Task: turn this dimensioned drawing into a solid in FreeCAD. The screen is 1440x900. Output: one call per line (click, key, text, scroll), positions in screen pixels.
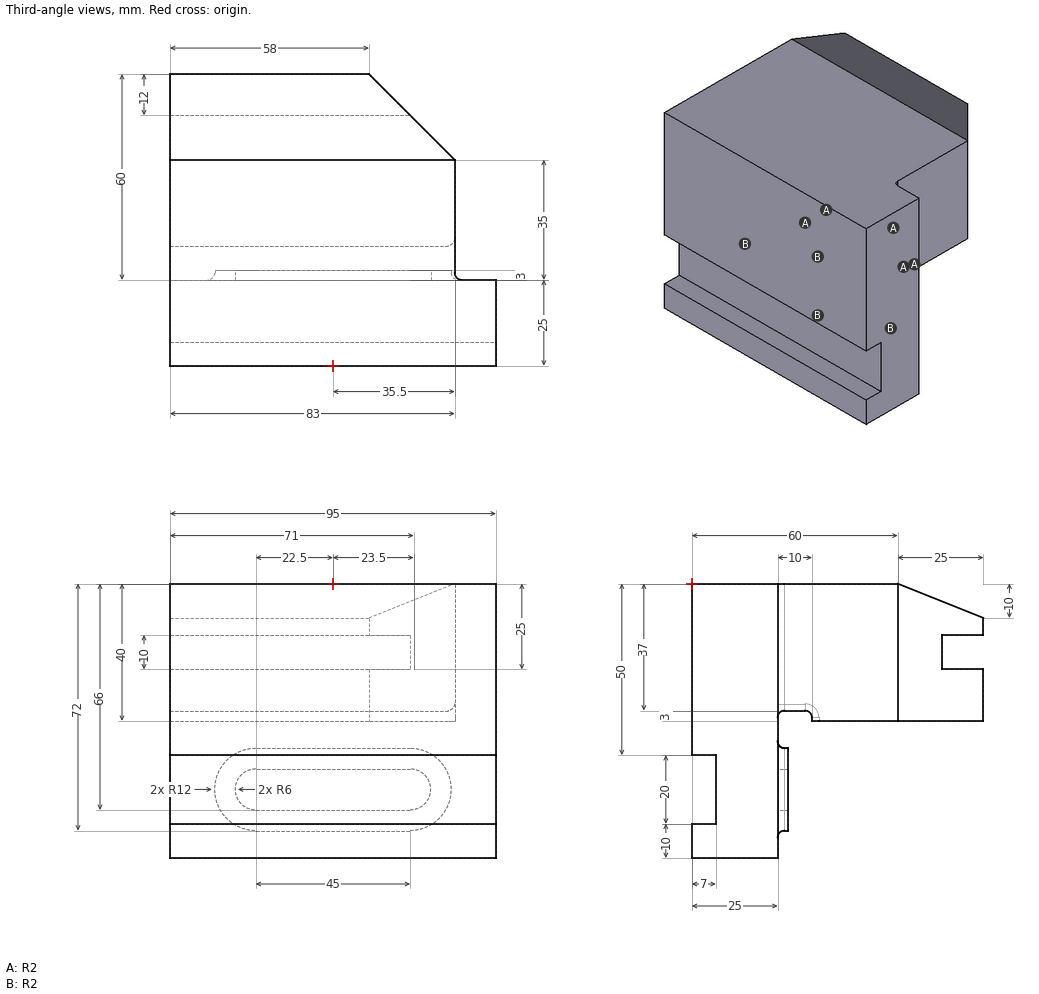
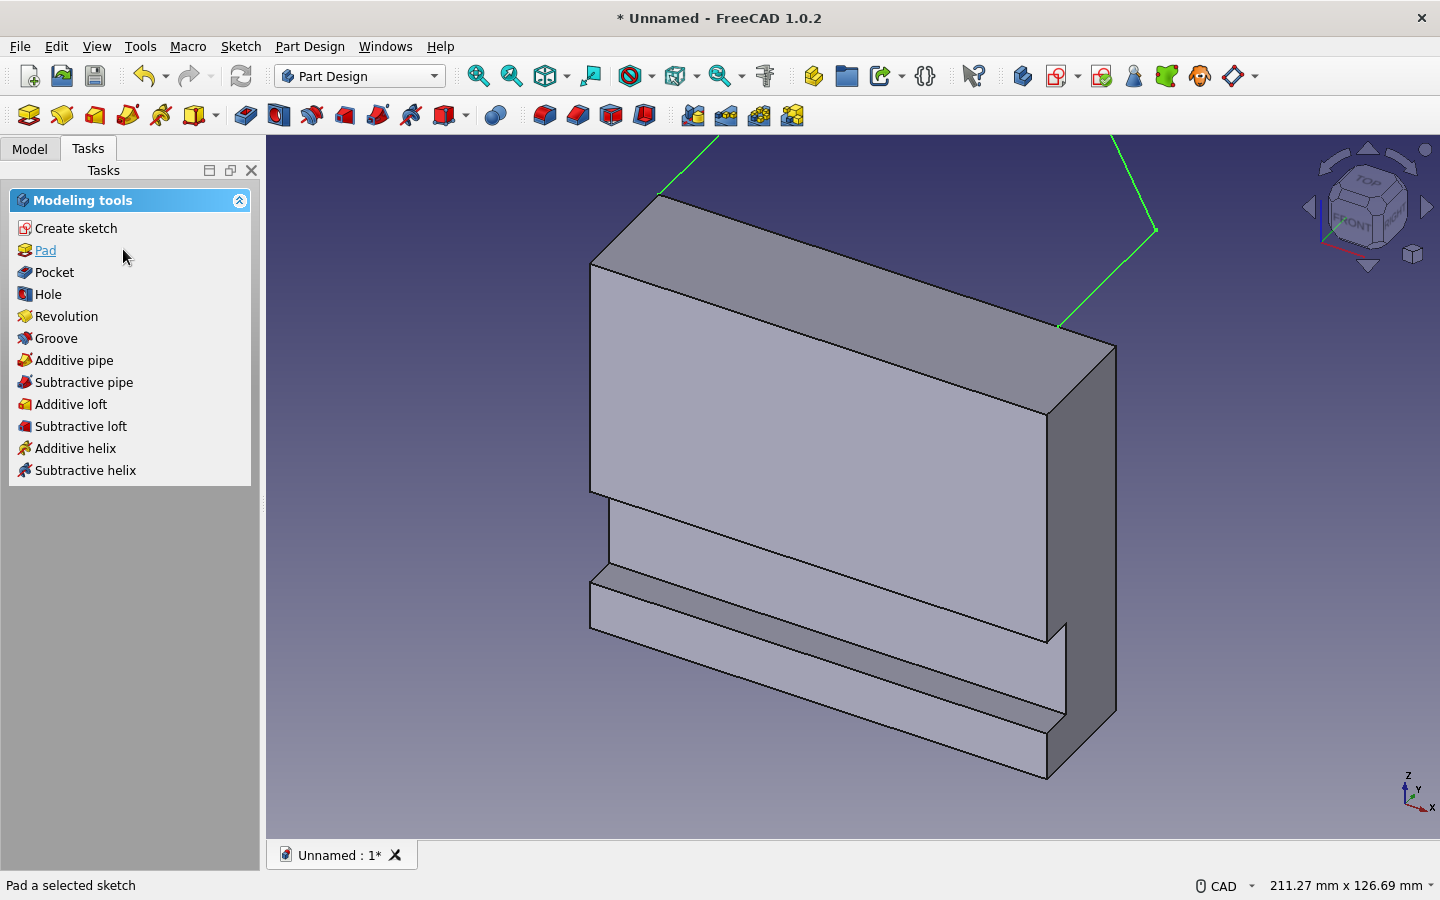
click(29, 116)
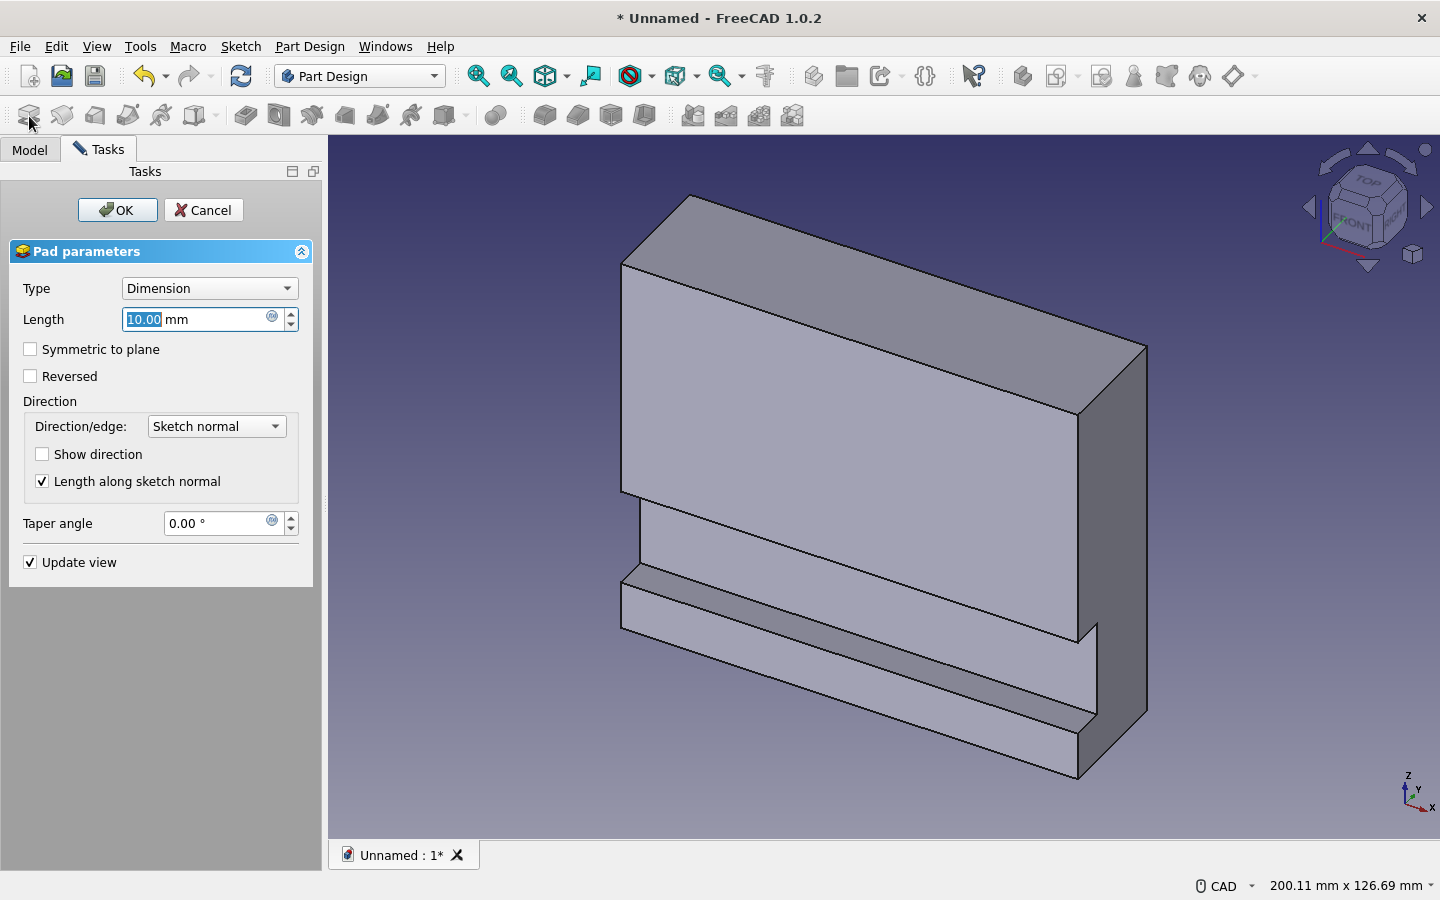
text(40)
key(Tab)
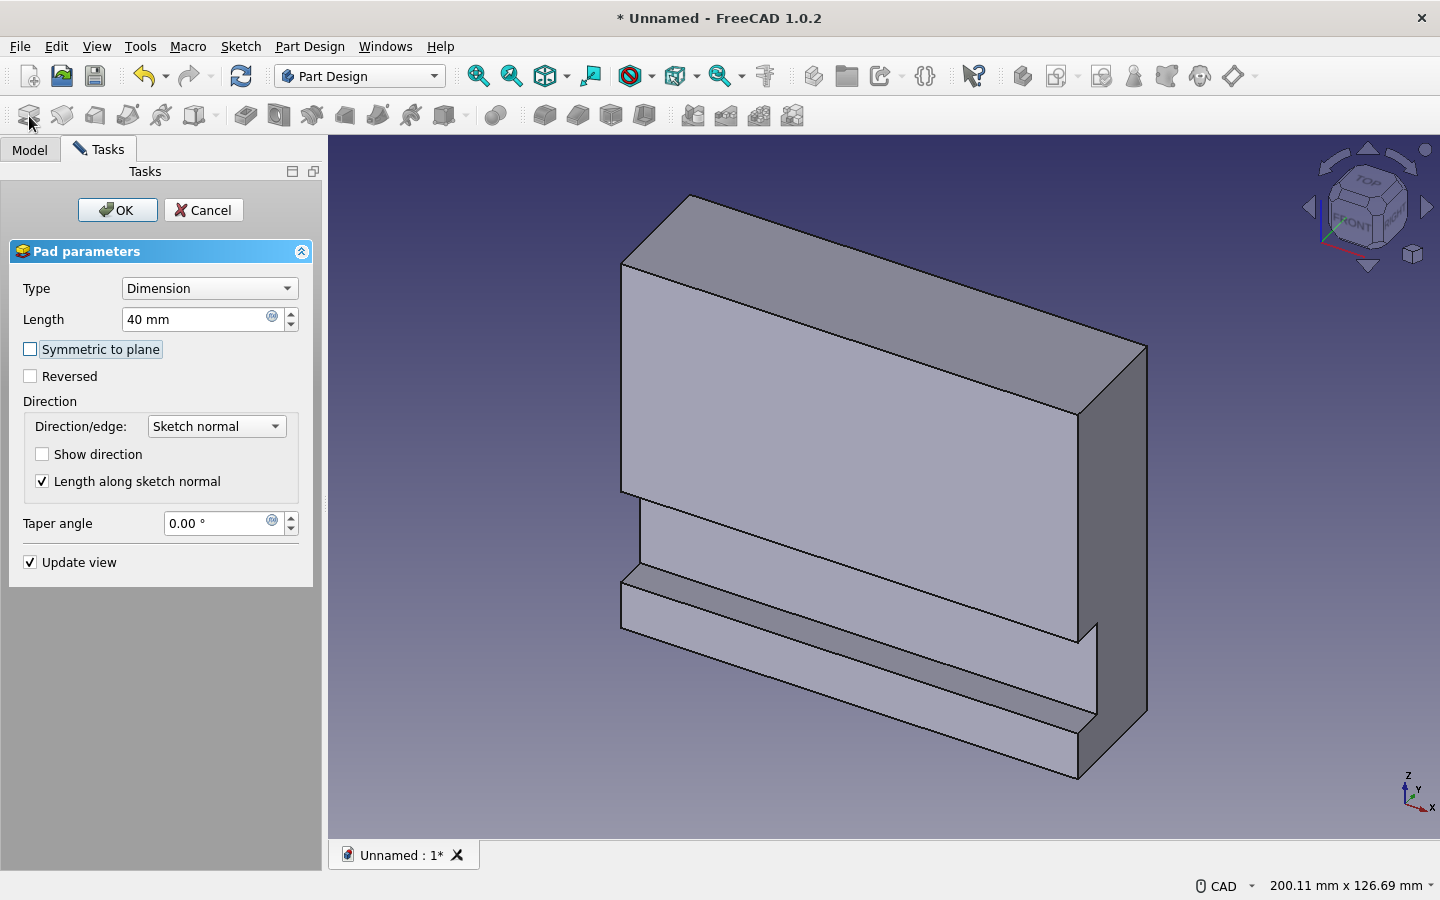
click(31, 376)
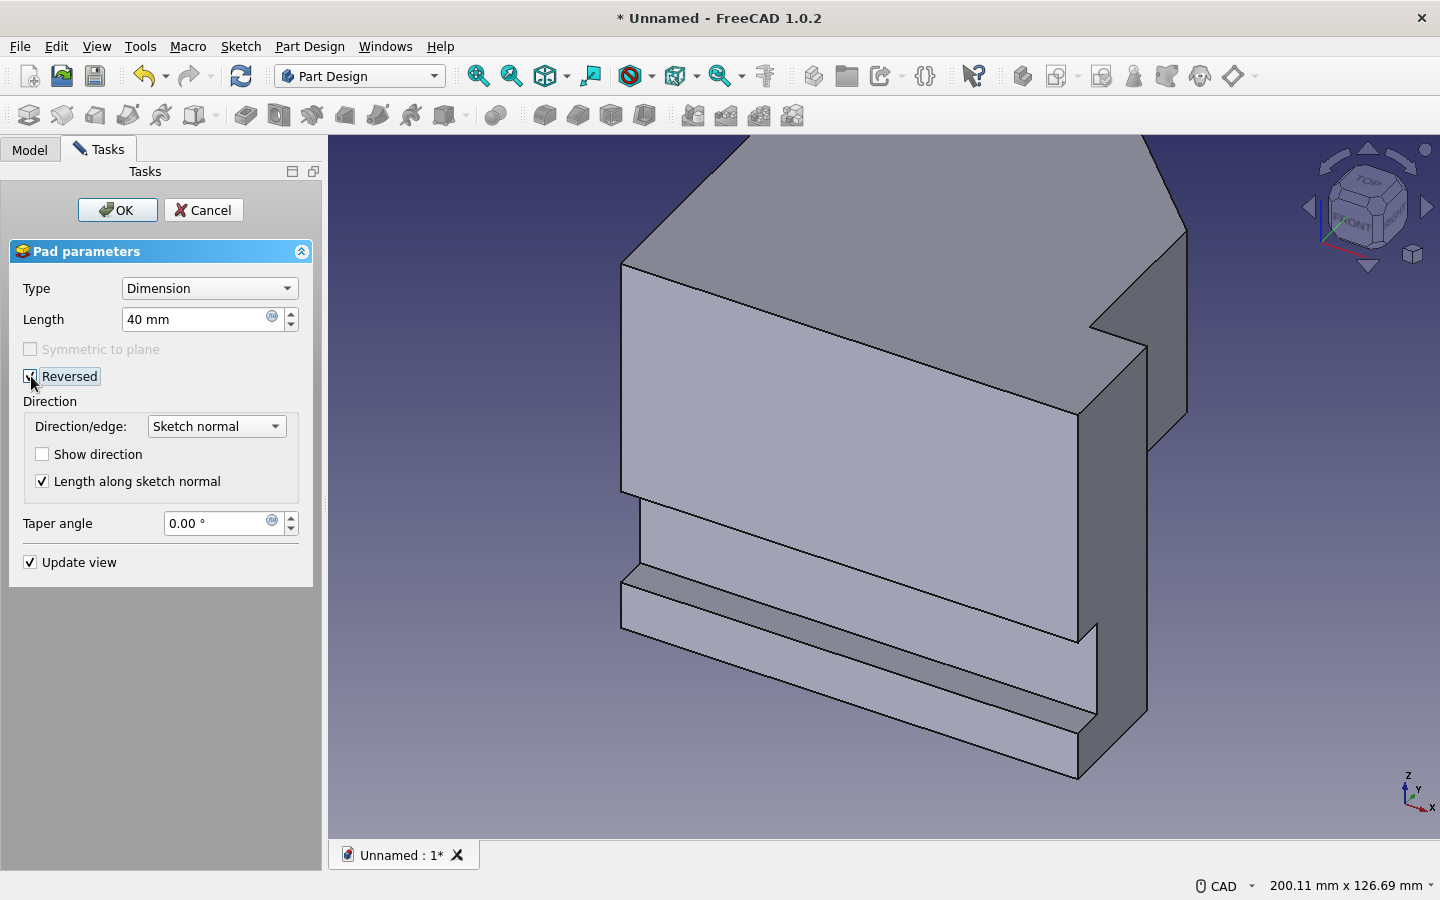
click(118, 210)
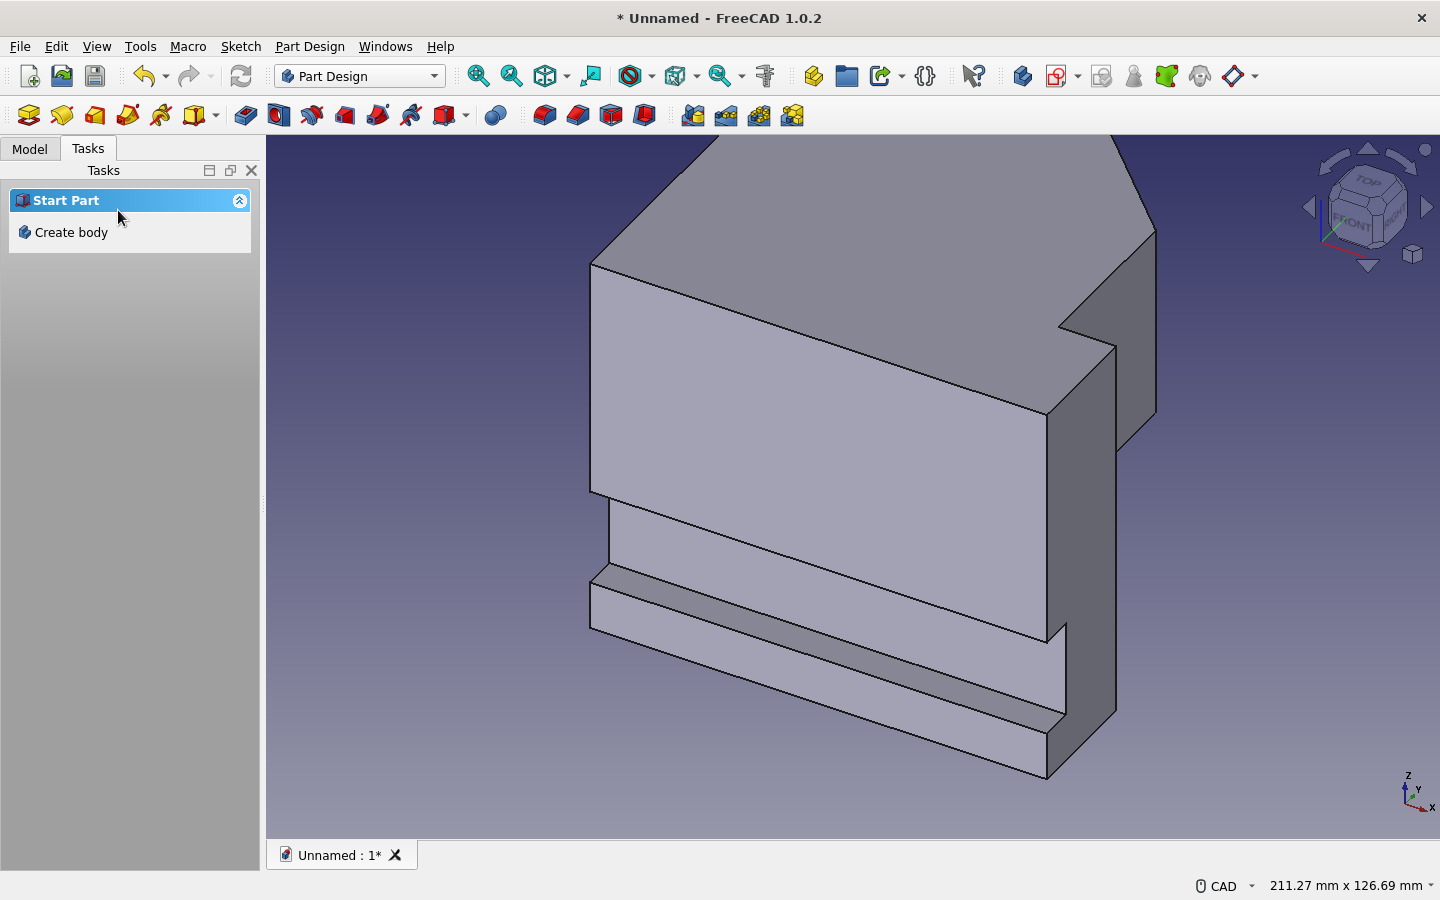
click(479, 76)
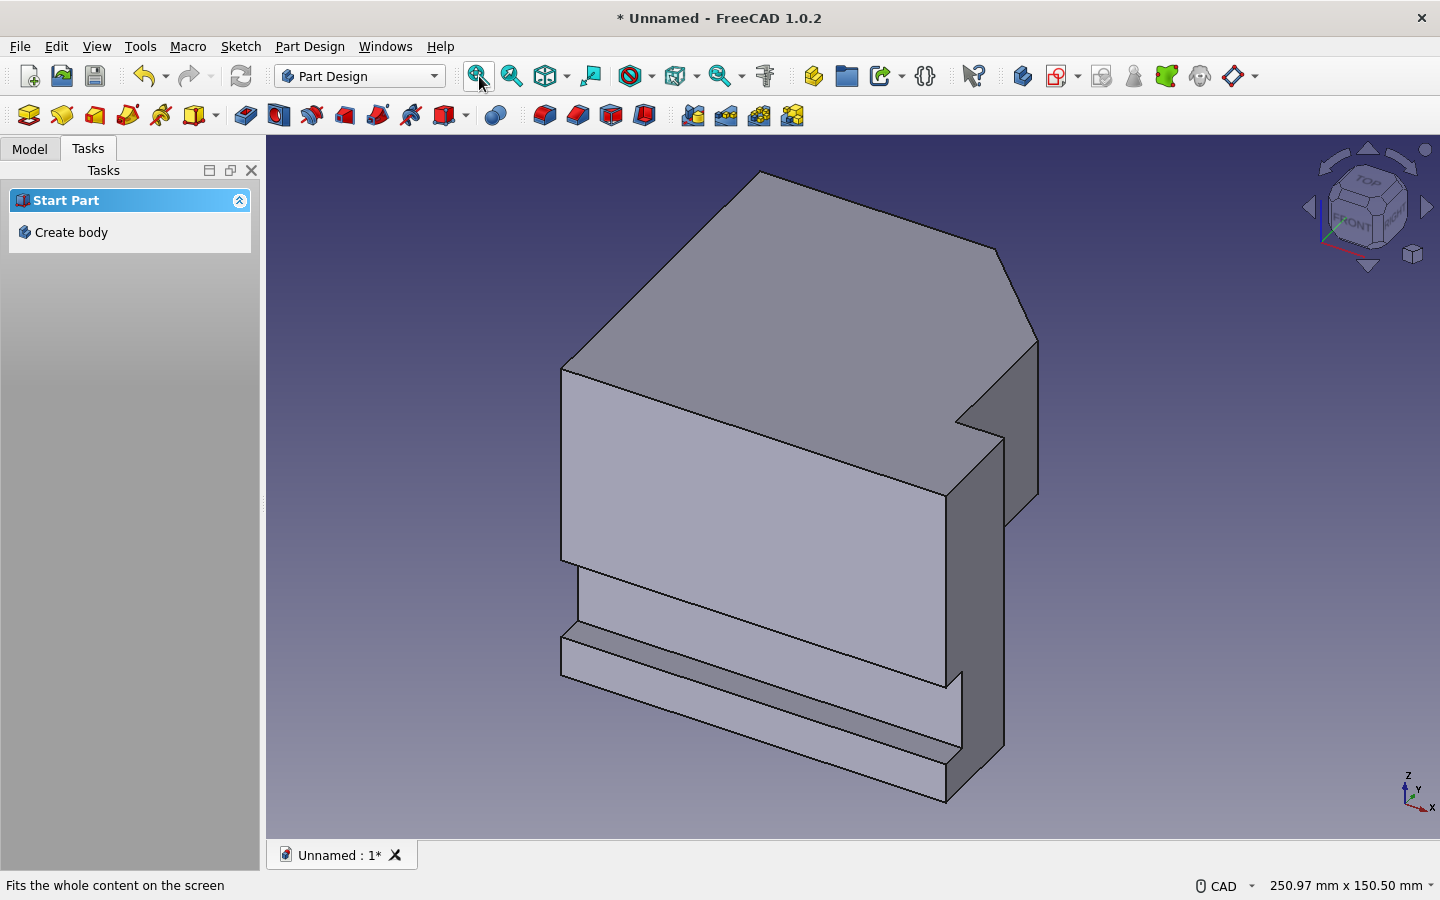
click(1009, 423)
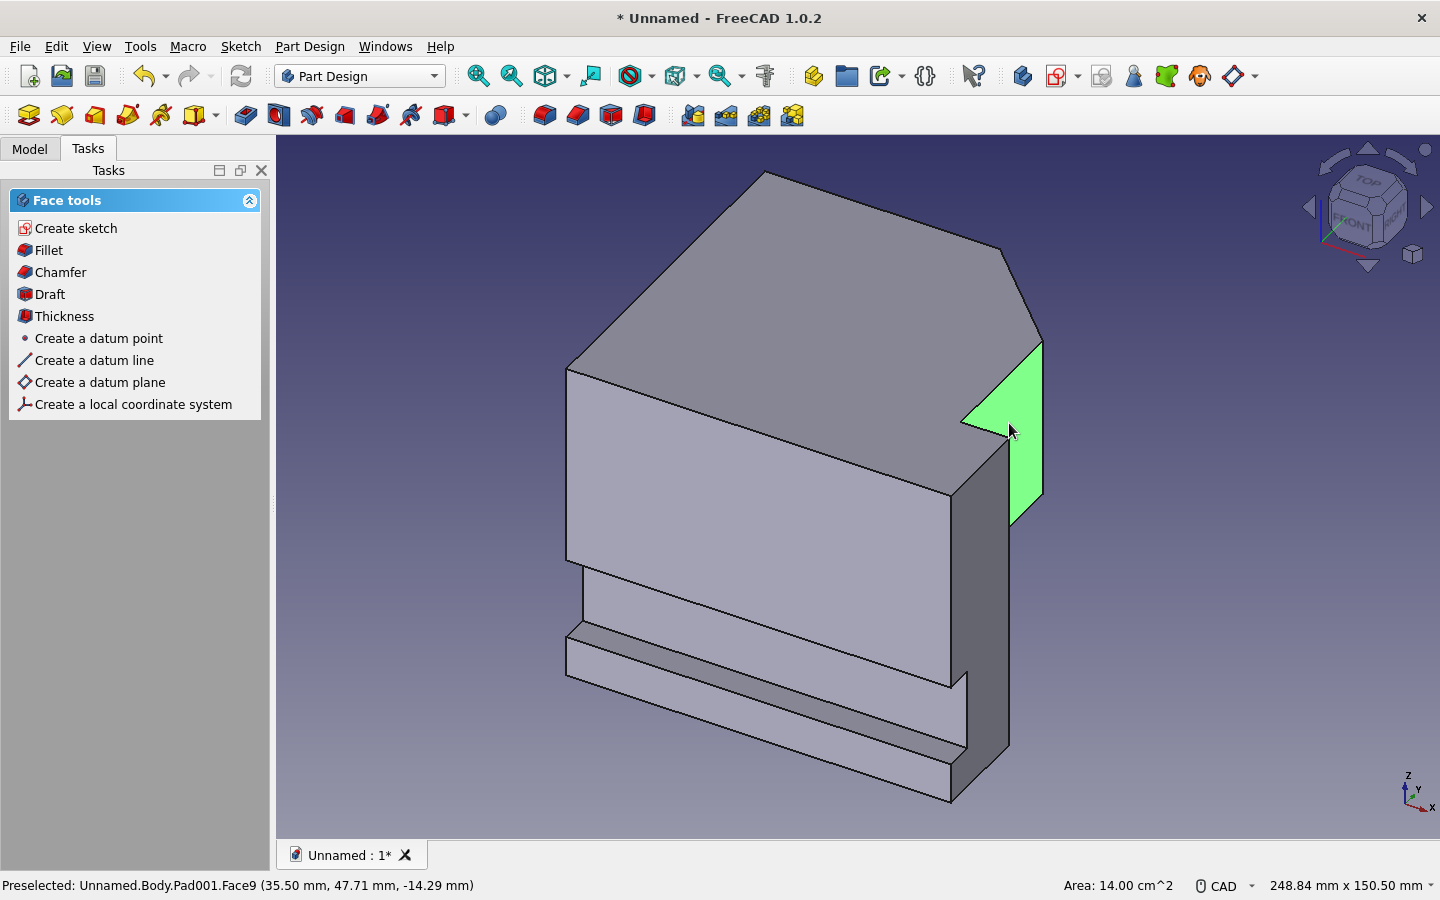
click(1056, 76)